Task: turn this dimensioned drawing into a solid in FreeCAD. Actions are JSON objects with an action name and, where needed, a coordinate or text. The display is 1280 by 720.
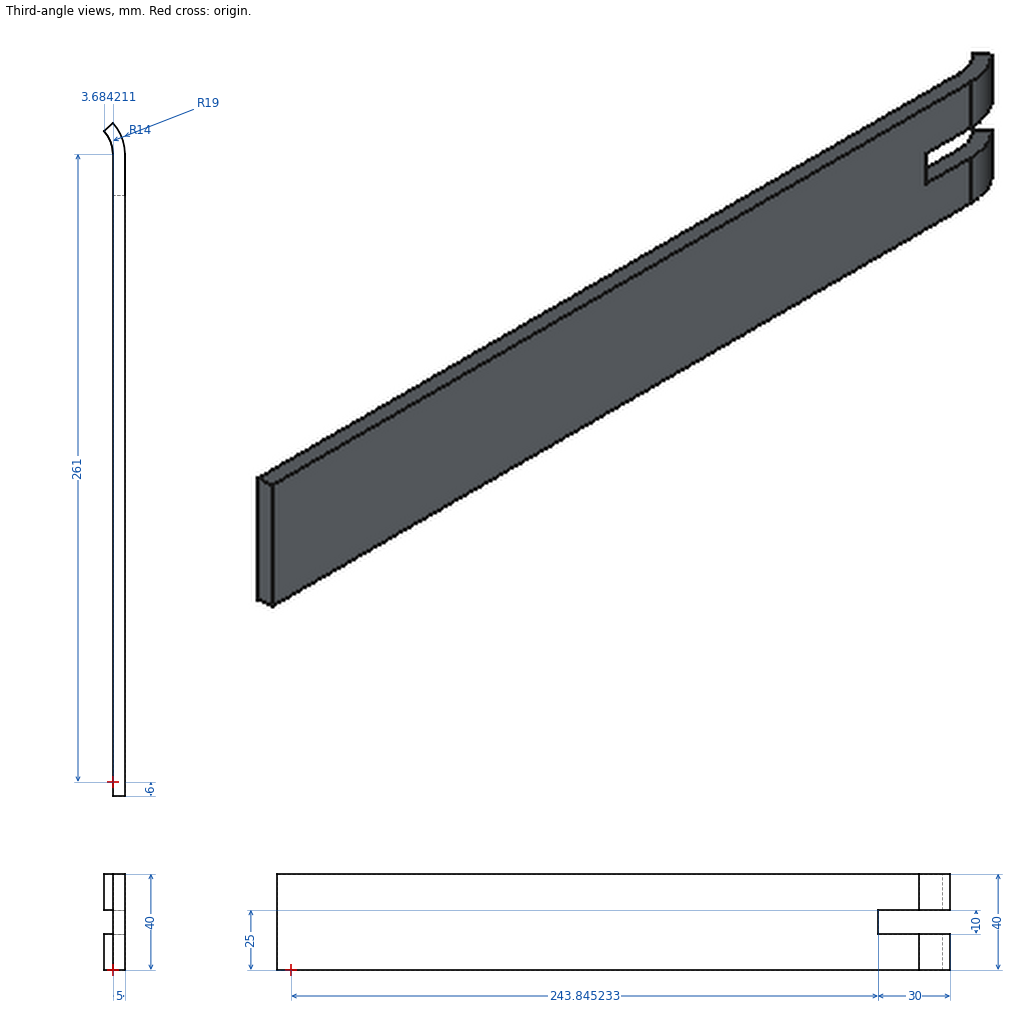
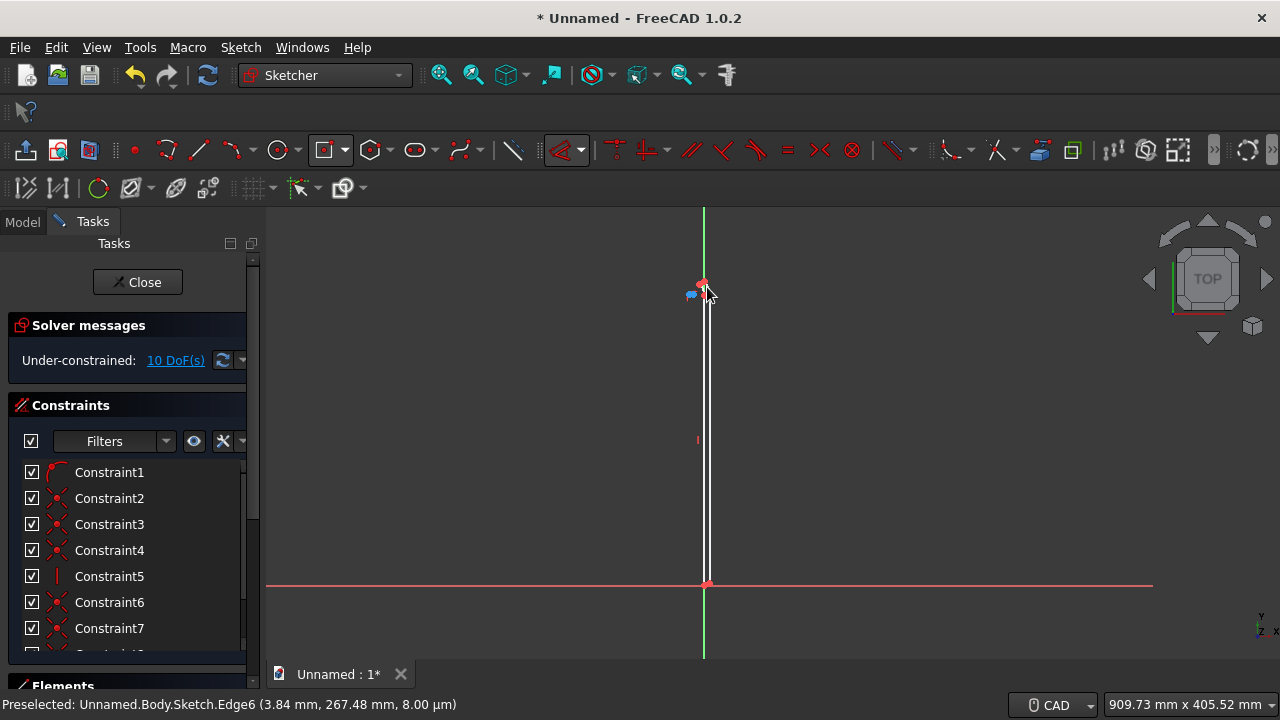
{"action": "scroll", "coordinate": [704, 383], "scroll_direction": "up", "scroll_amount": 5}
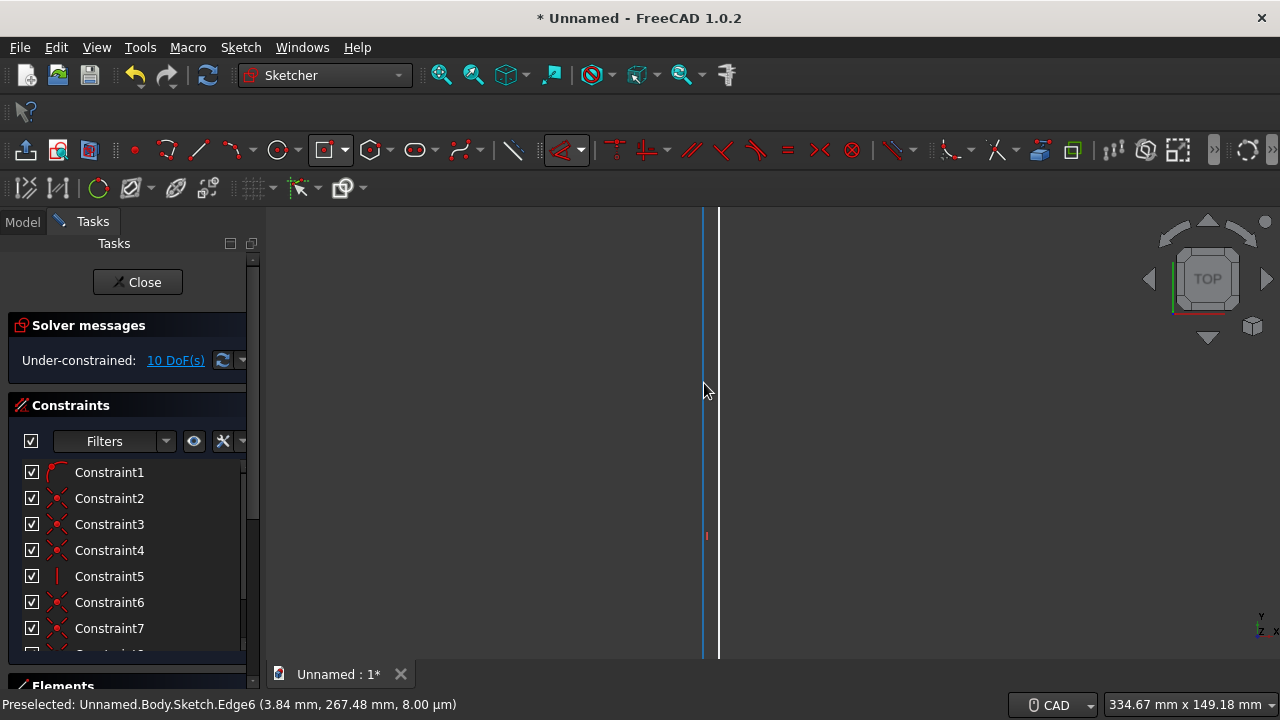
{"action": "left_click", "coordinate": [703, 381]}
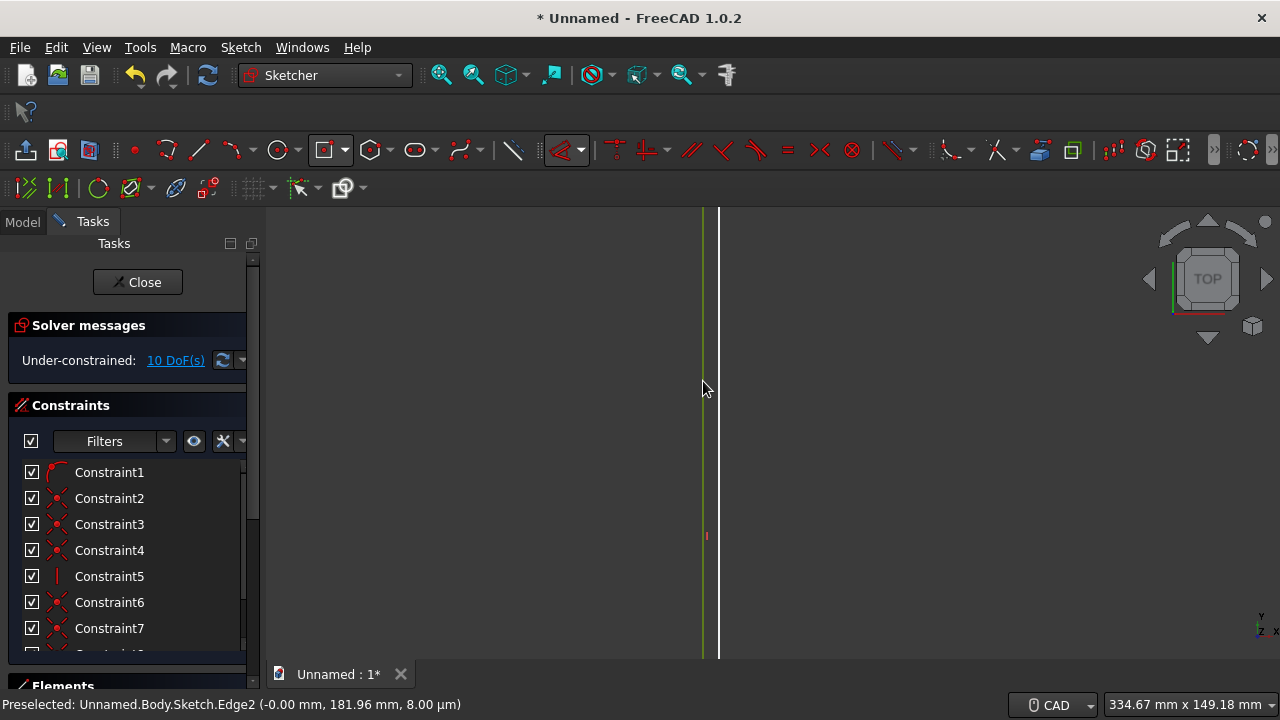
{"action": "scroll", "coordinate": [704, 383], "scroll_direction": "down", "scroll_amount": 5}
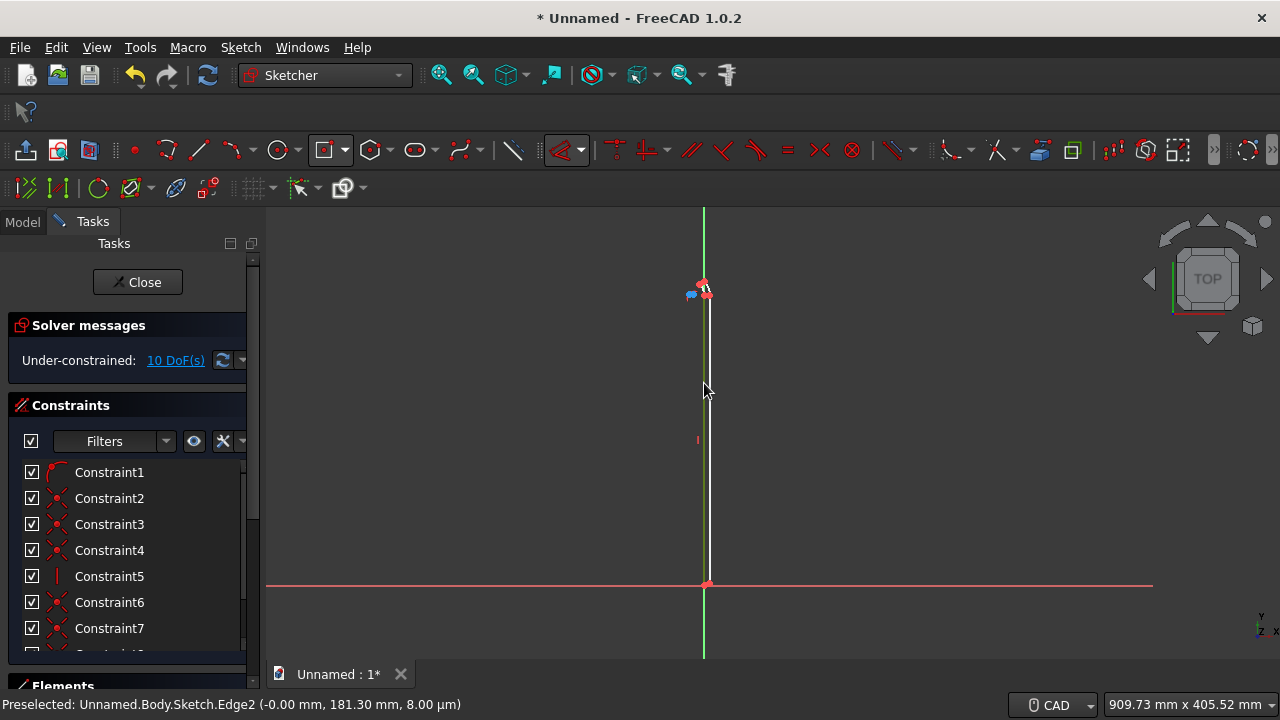
{"action": "scroll", "coordinate": [704, 292], "scroll_direction": "up", "scroll_amount": 7}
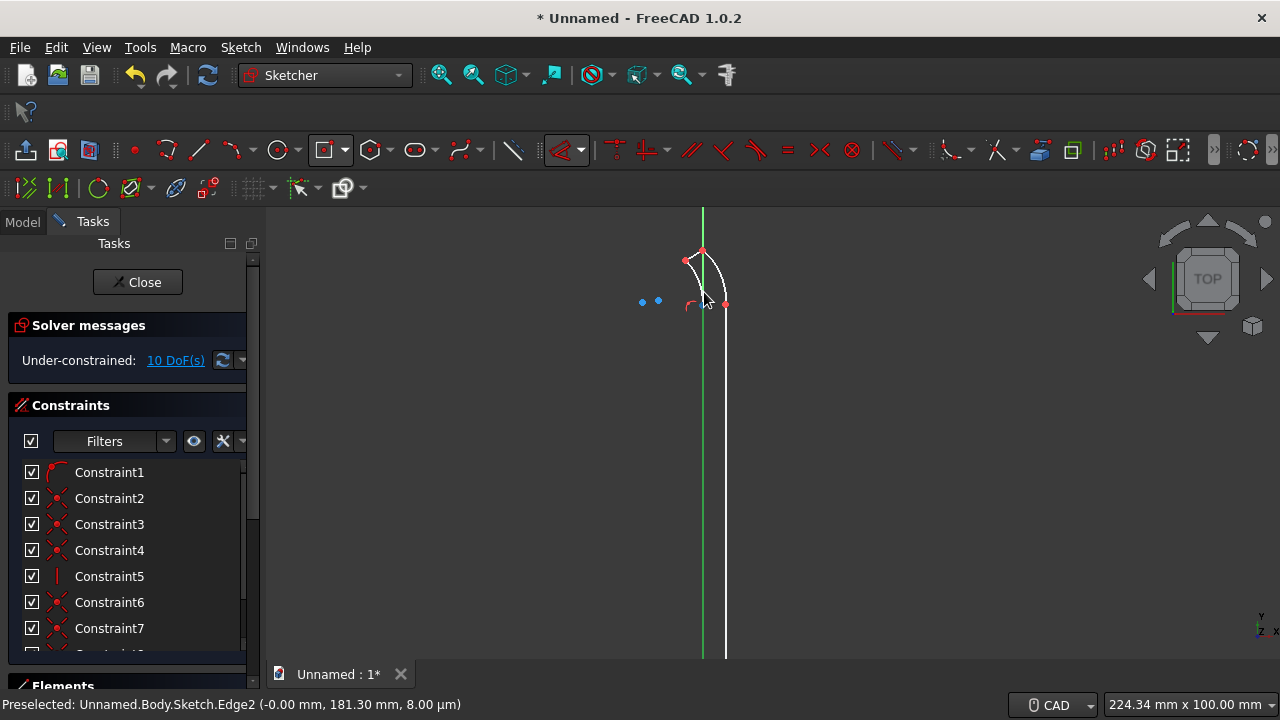
{"action": "left_click", "coordinate": [702, 291]}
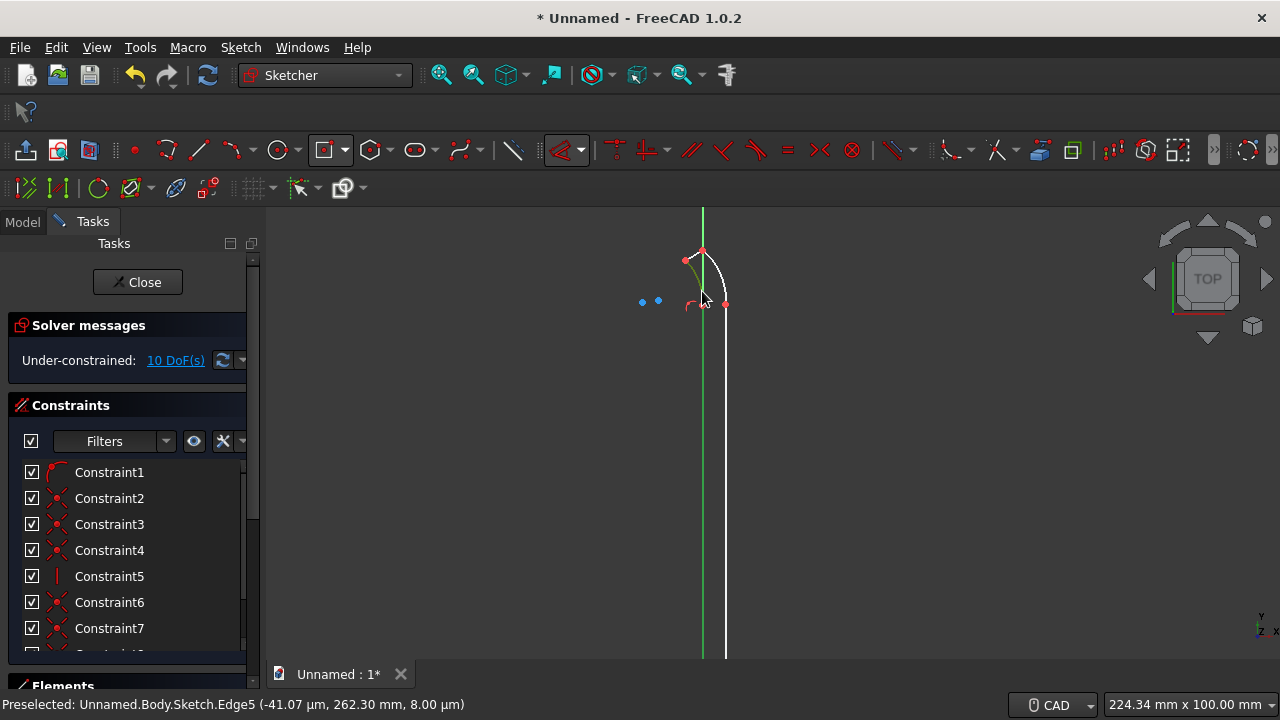
{"action": "left_click", "coordinate": [756, 150]}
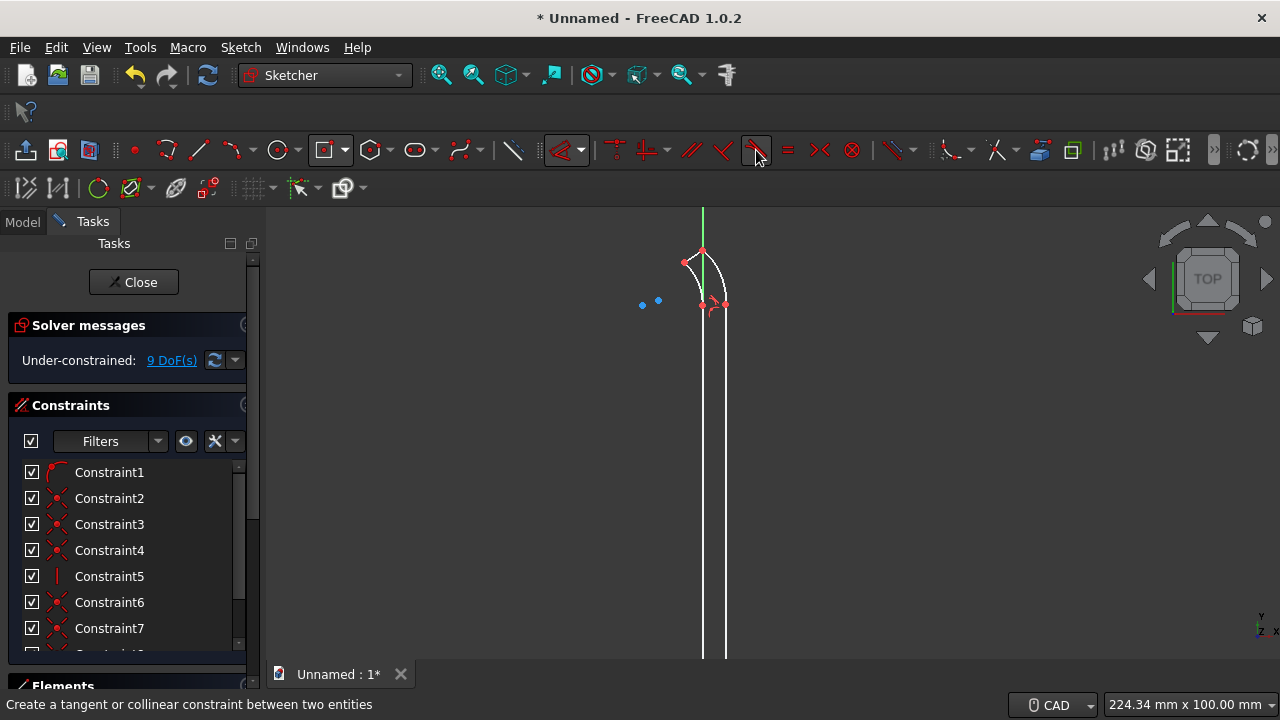
{"action": "left_click", "coordinate": [726, 538]}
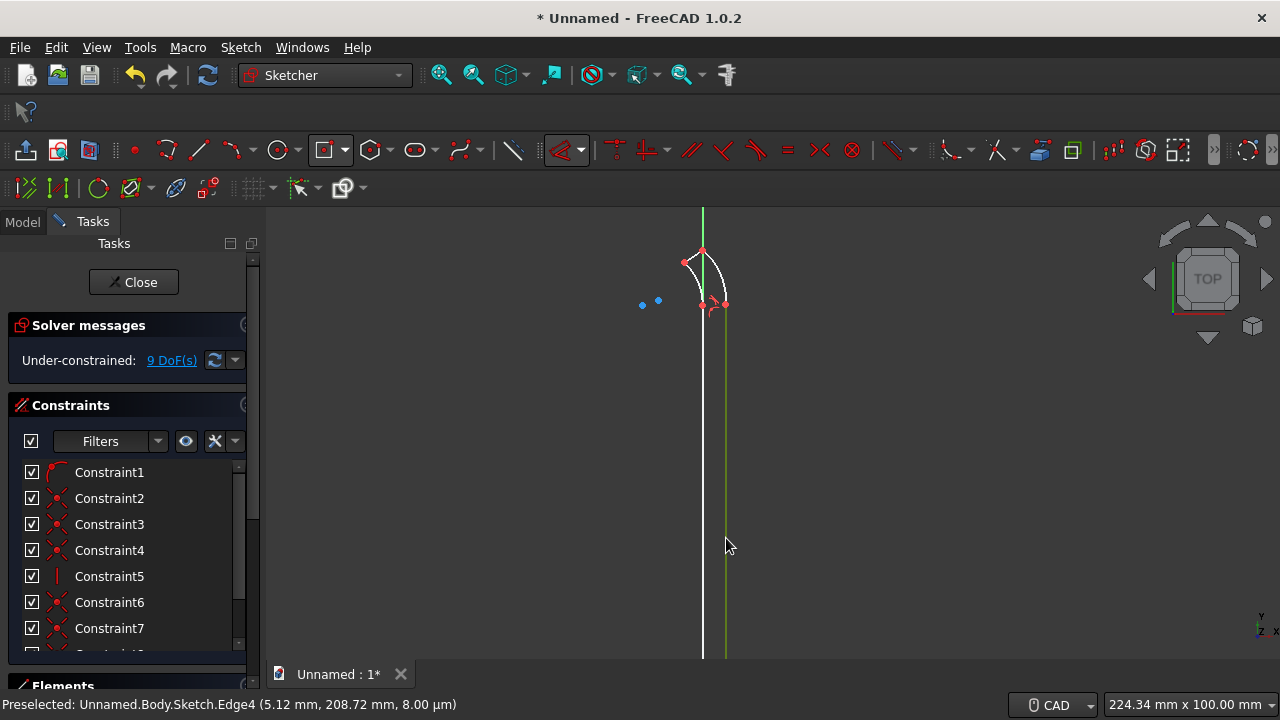
{"action": "left_click", "coordinate": [724, 286]}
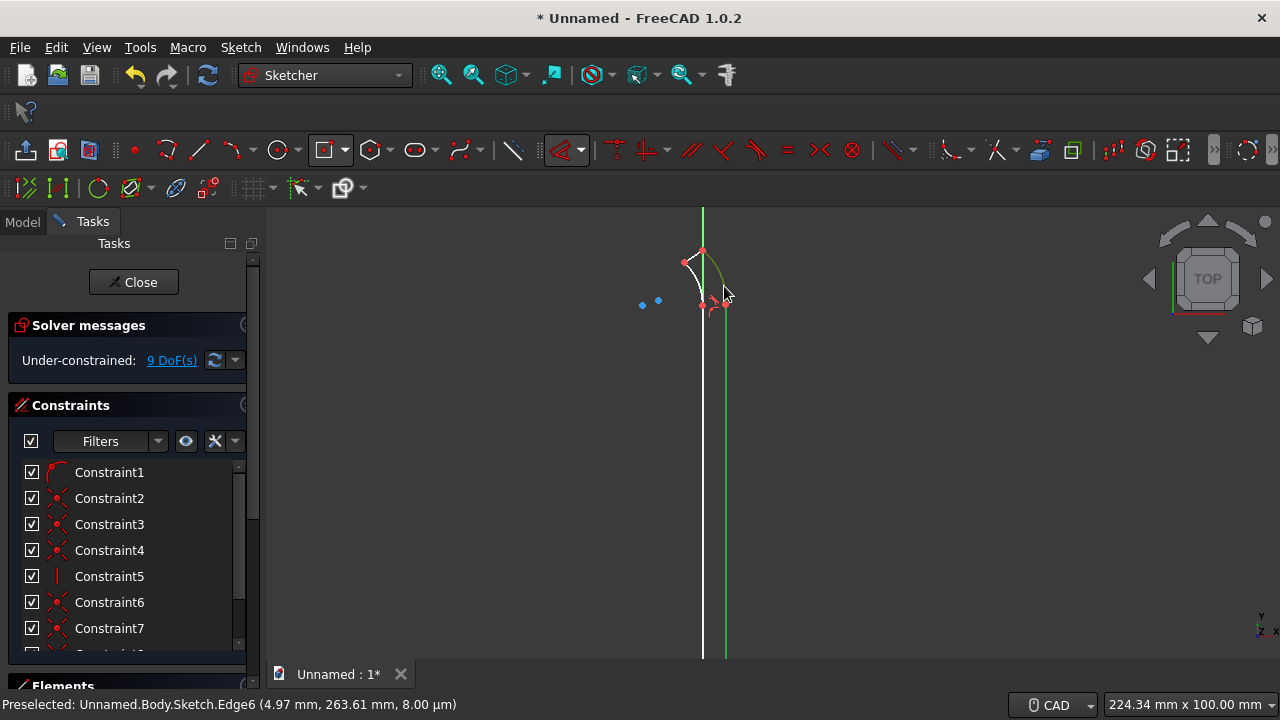
{"action": "left_click", "coordinate": [756, 150]}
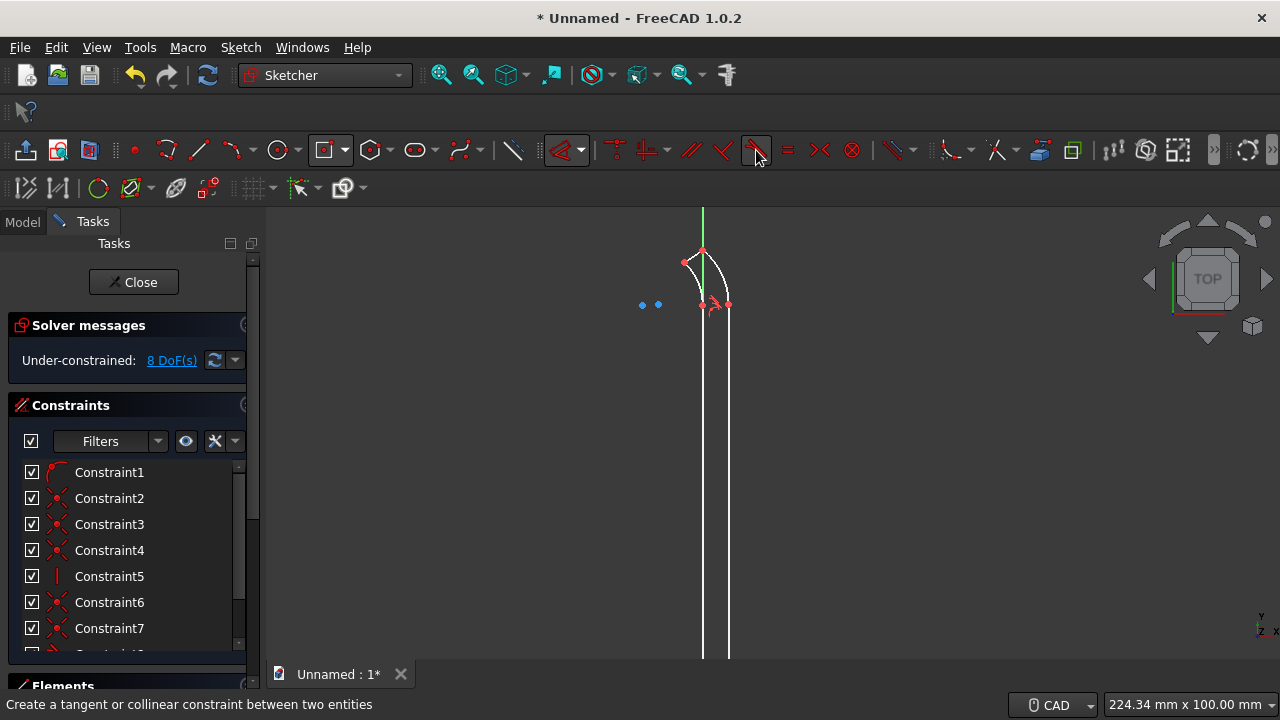
{"action": "scroll", "coordinate": [704, 292], "scroll_direction": "down", "scroll_amount": 7}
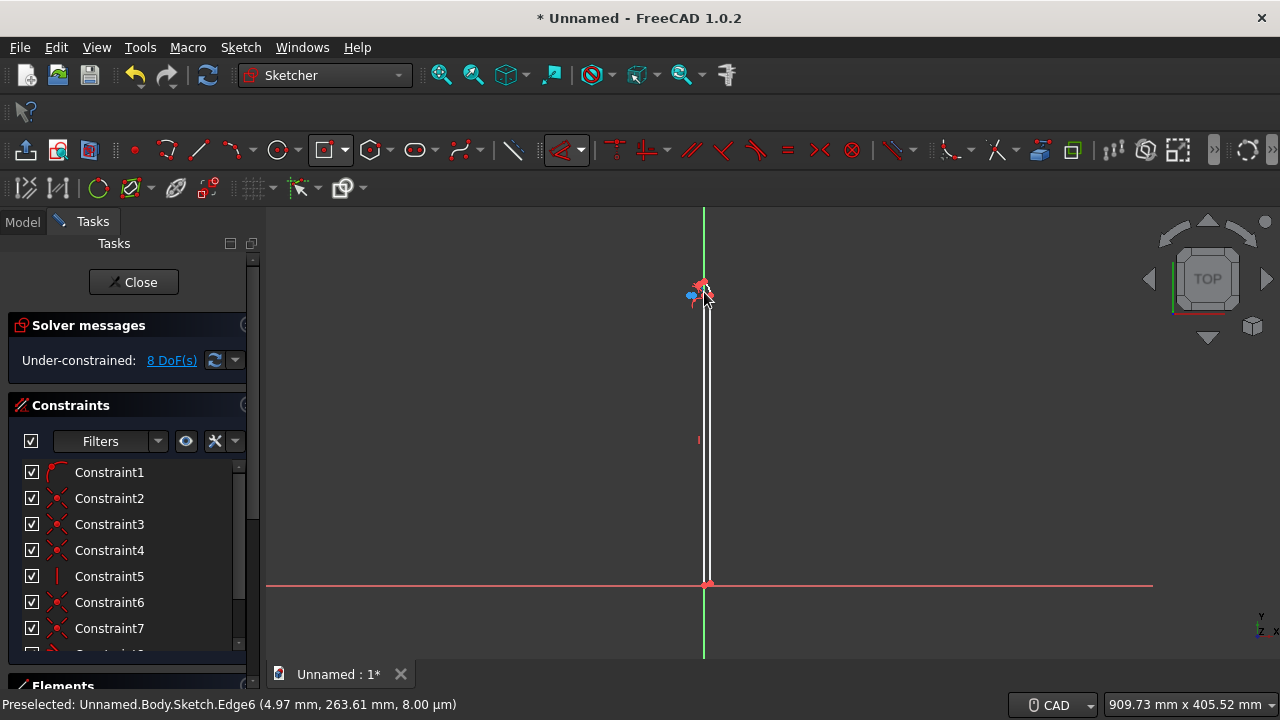
{"action": "scroll", "coordinate": [707, 585], "scroll_direction": "up", "scroll_amount": 9}